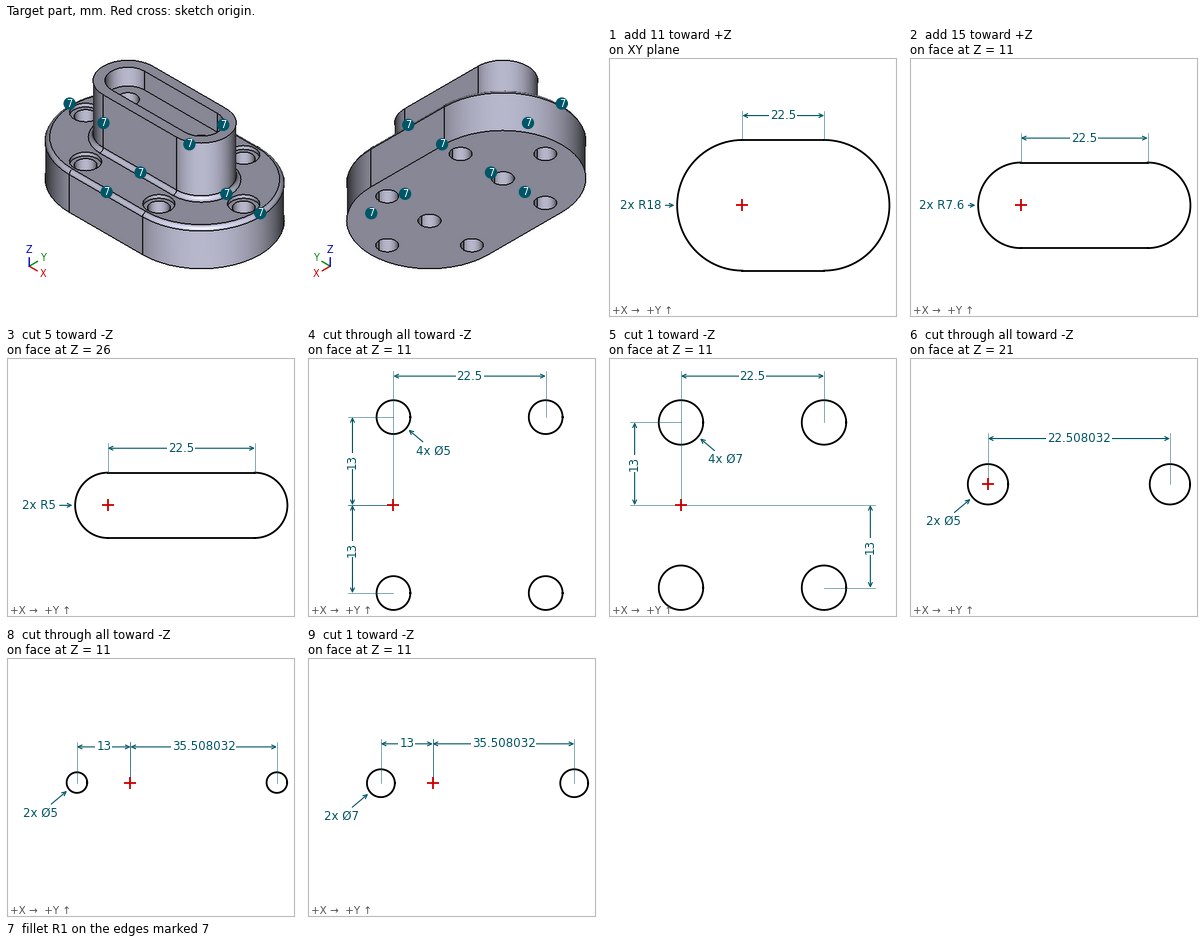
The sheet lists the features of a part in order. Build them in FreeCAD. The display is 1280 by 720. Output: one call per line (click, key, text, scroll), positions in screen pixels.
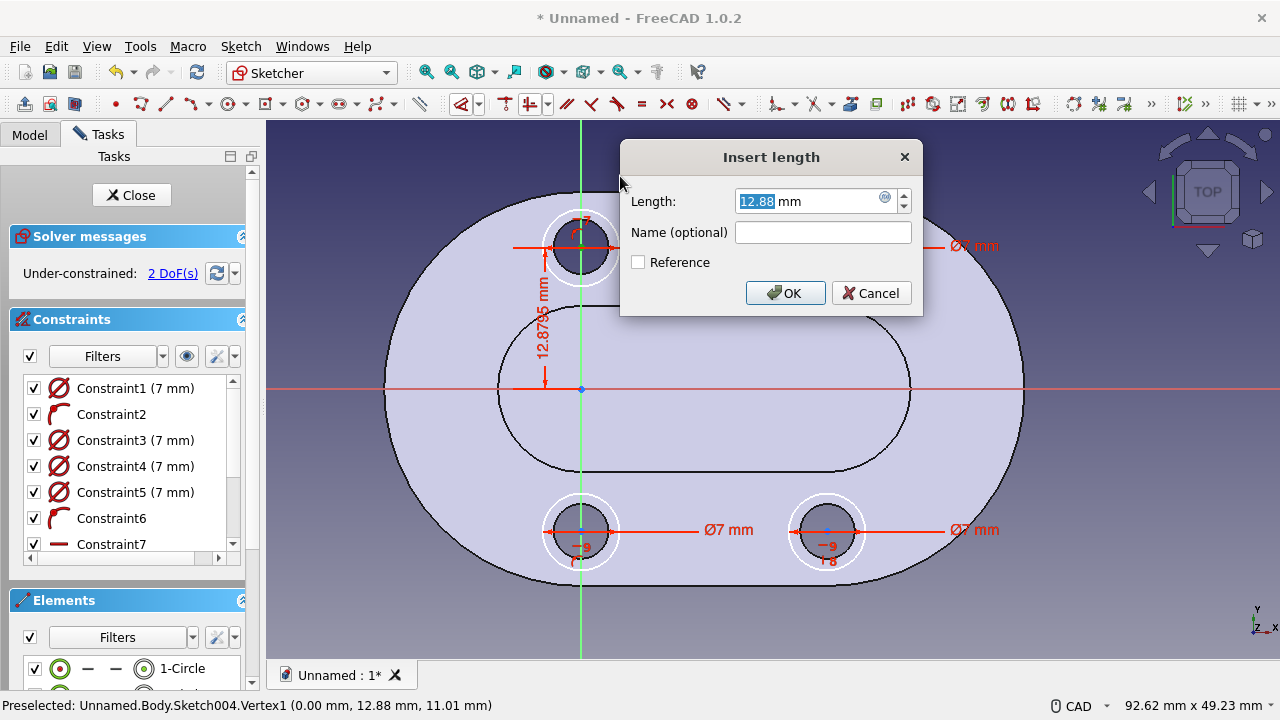
text(13)
key(Return)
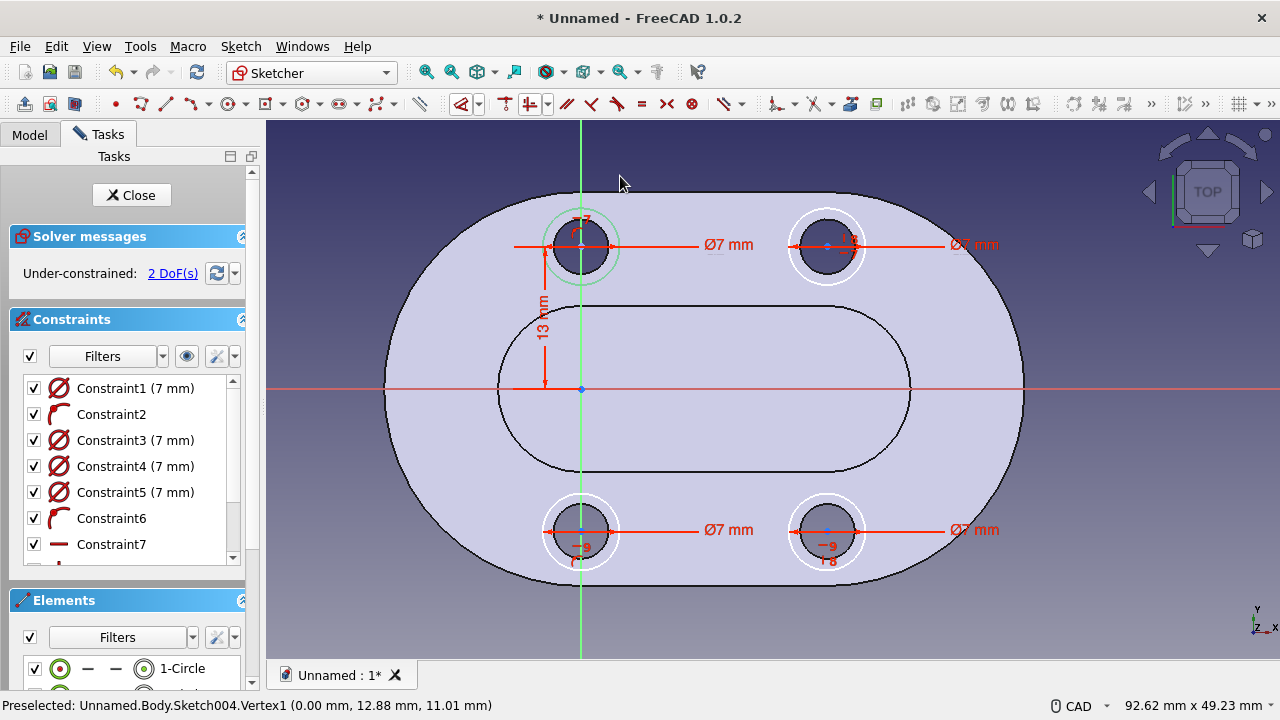
click(827, 532)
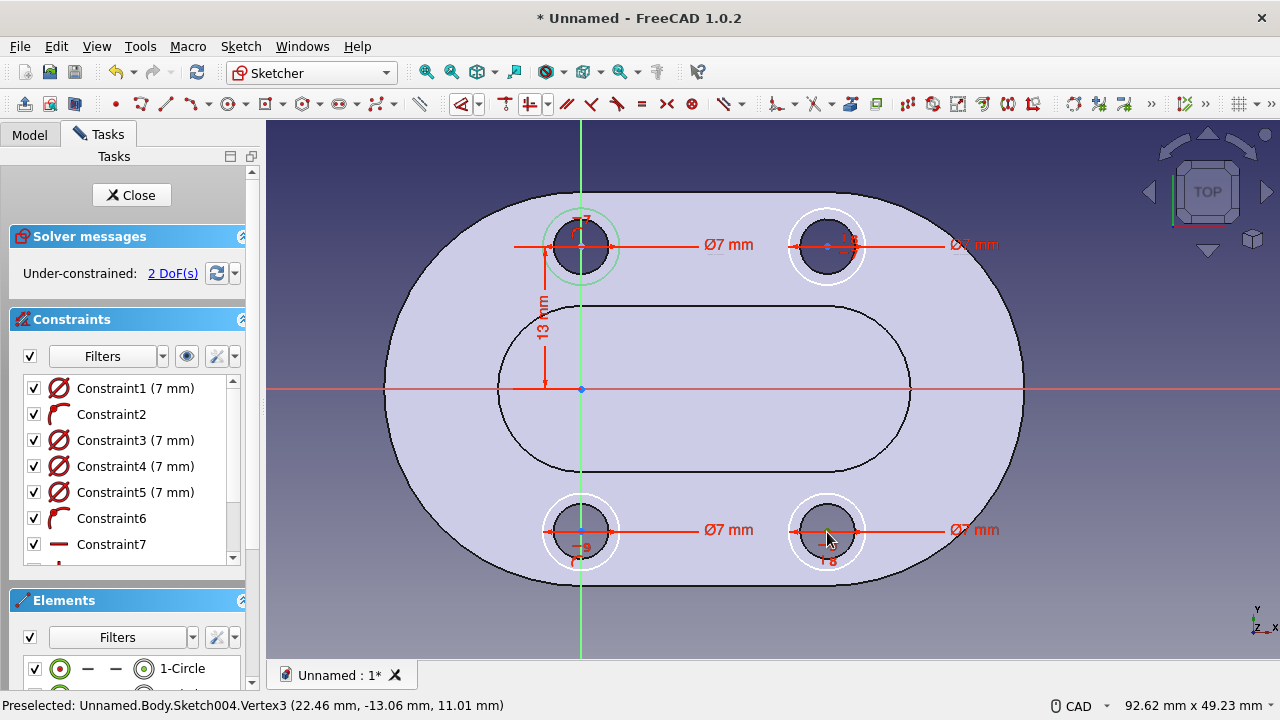
key(i)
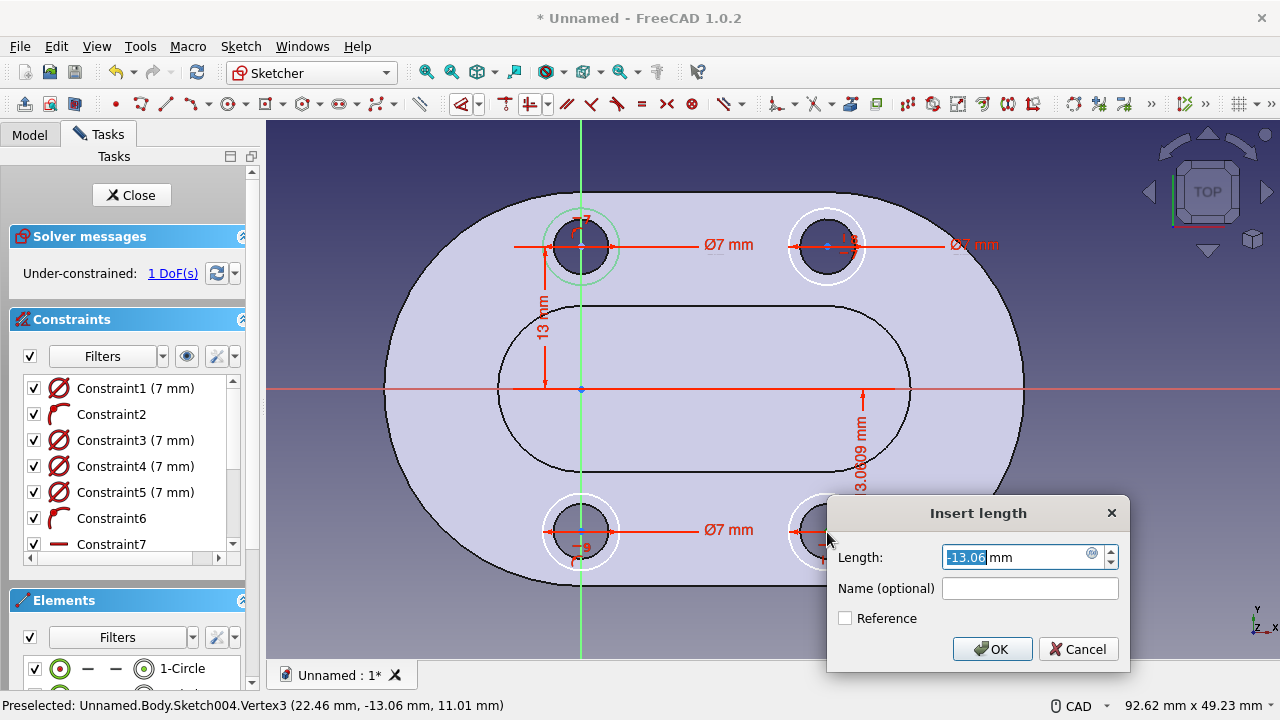
text(-13)
key(Return)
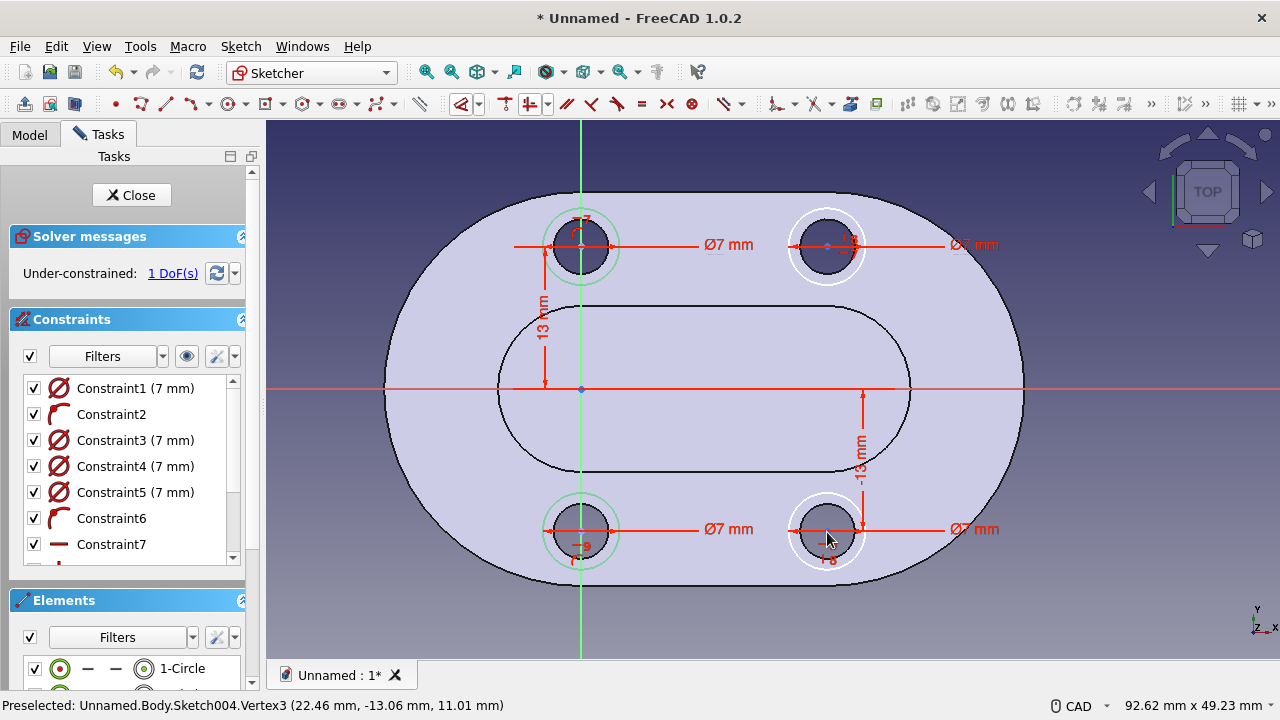
click(827, 247)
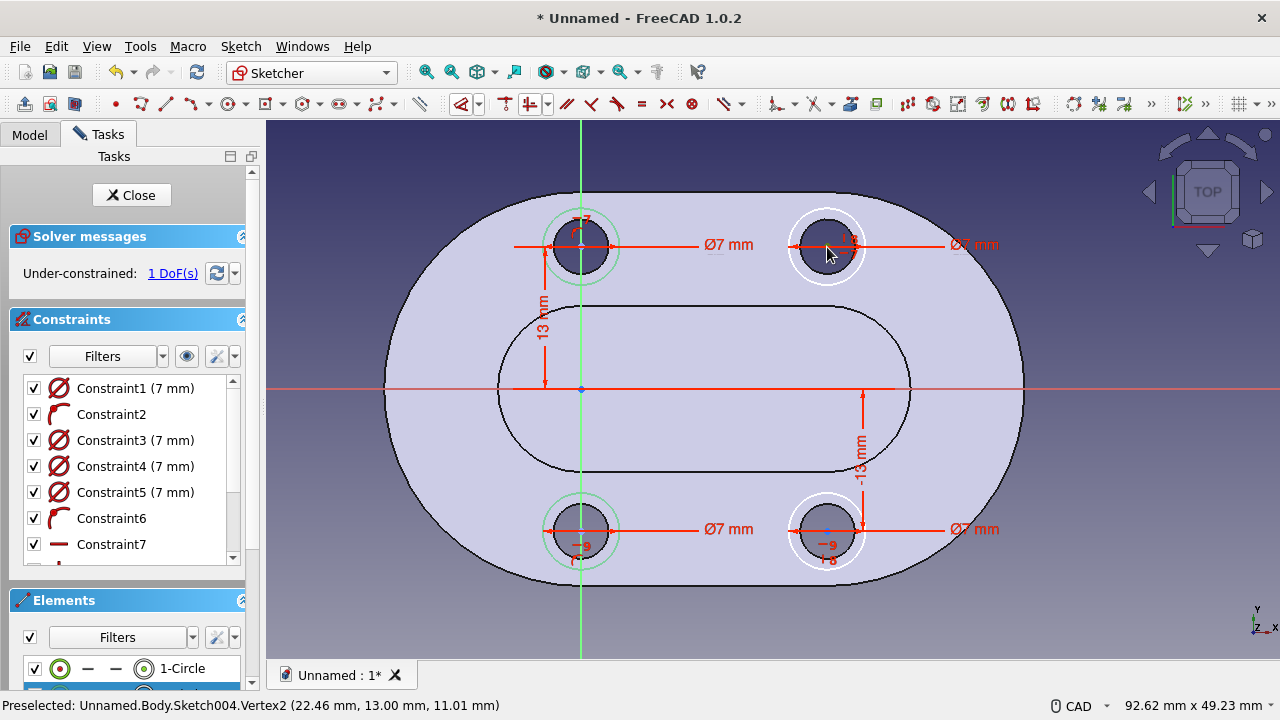
key(l)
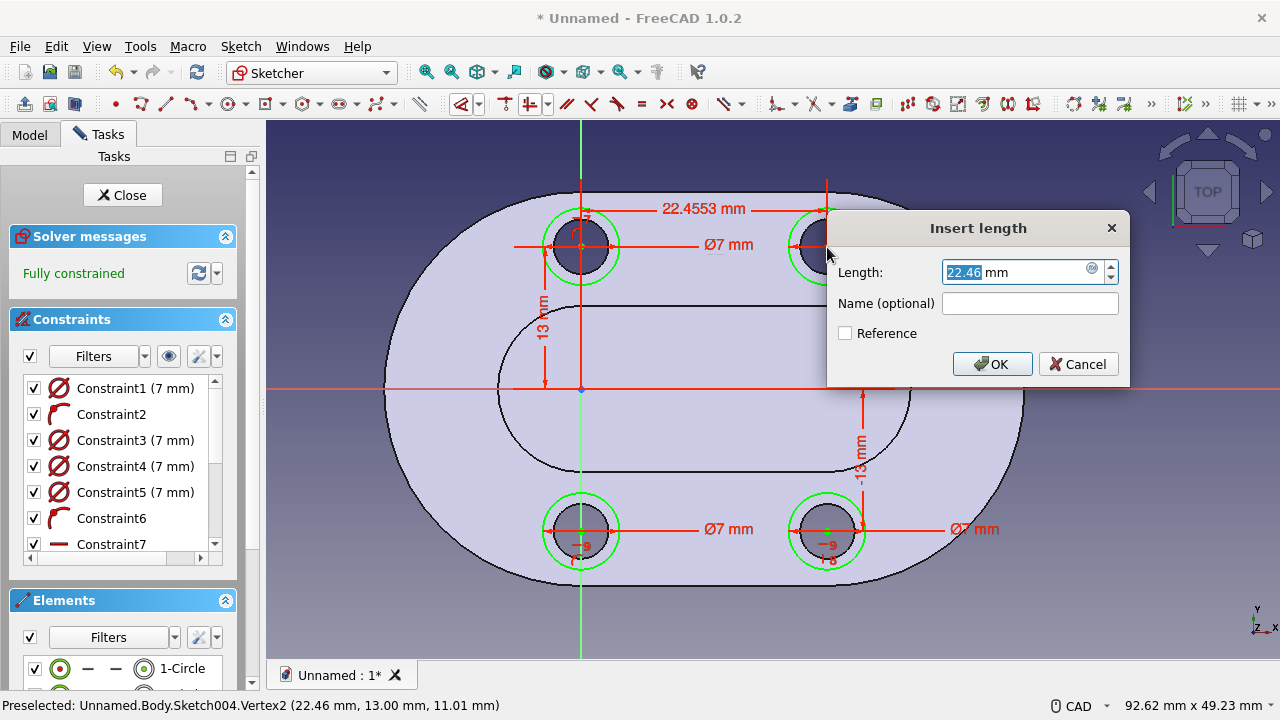
text(22.5)
key(Return)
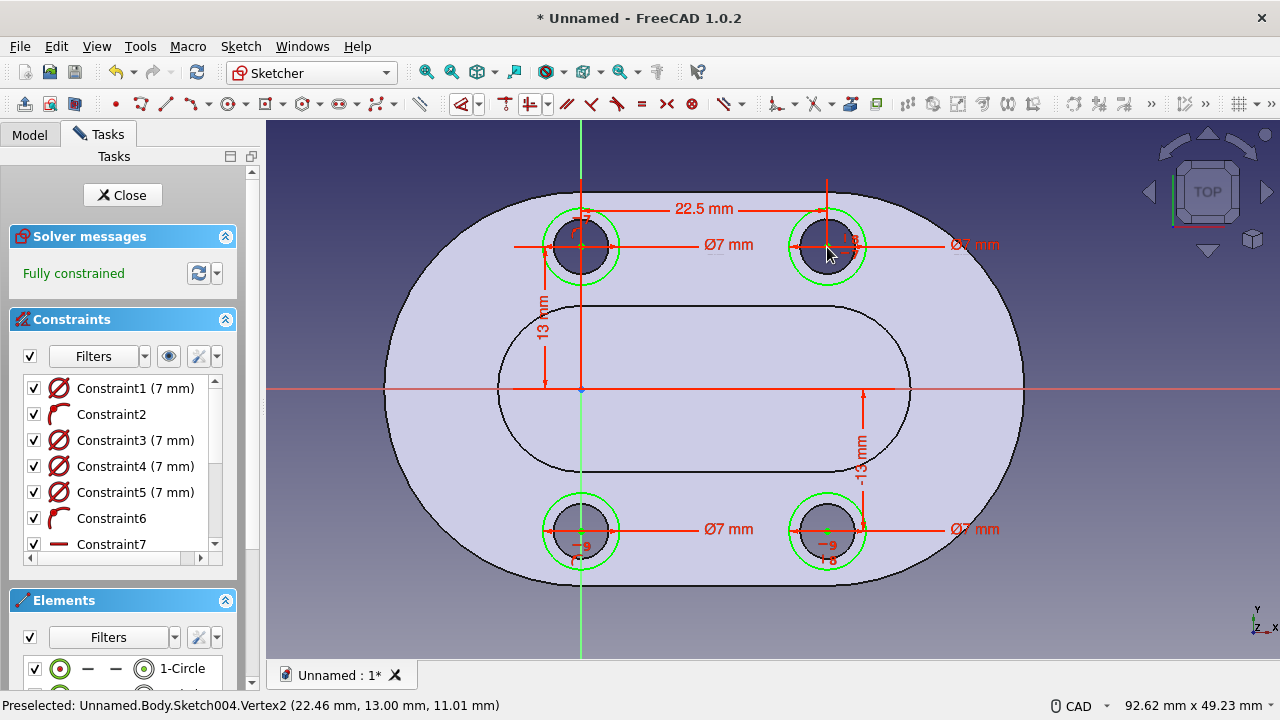
click(123, 195)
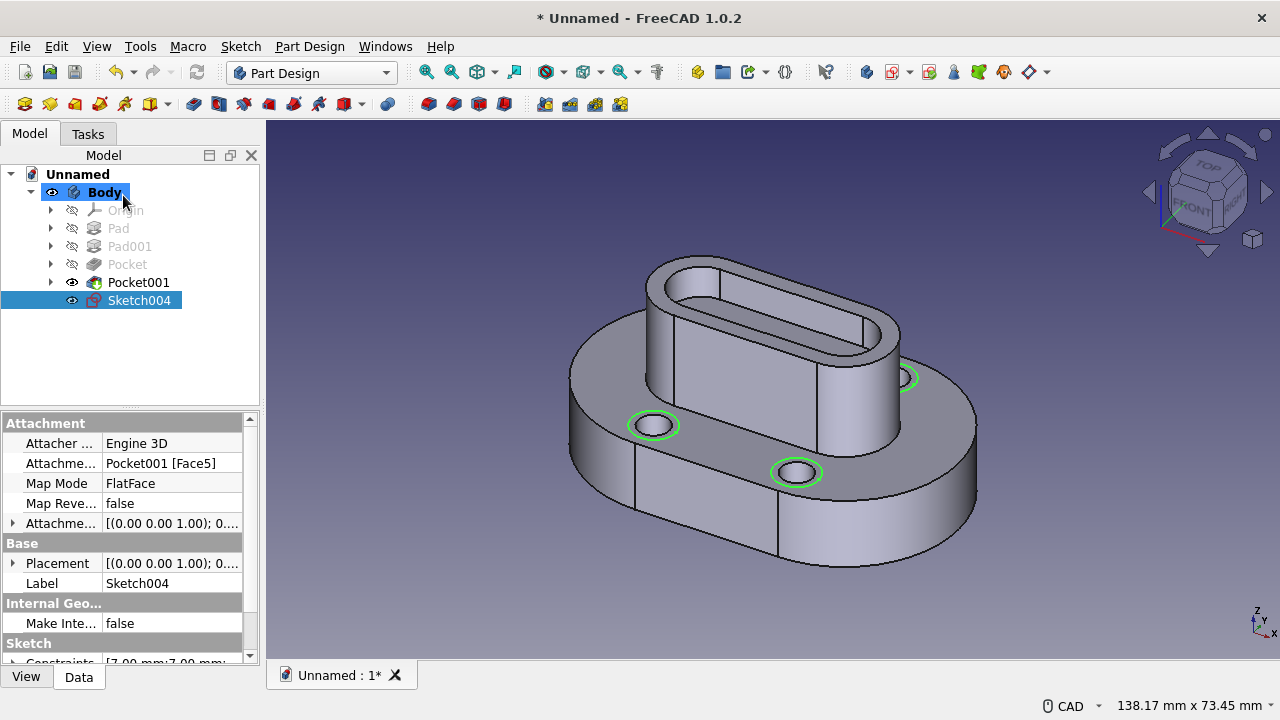
click(194, 104)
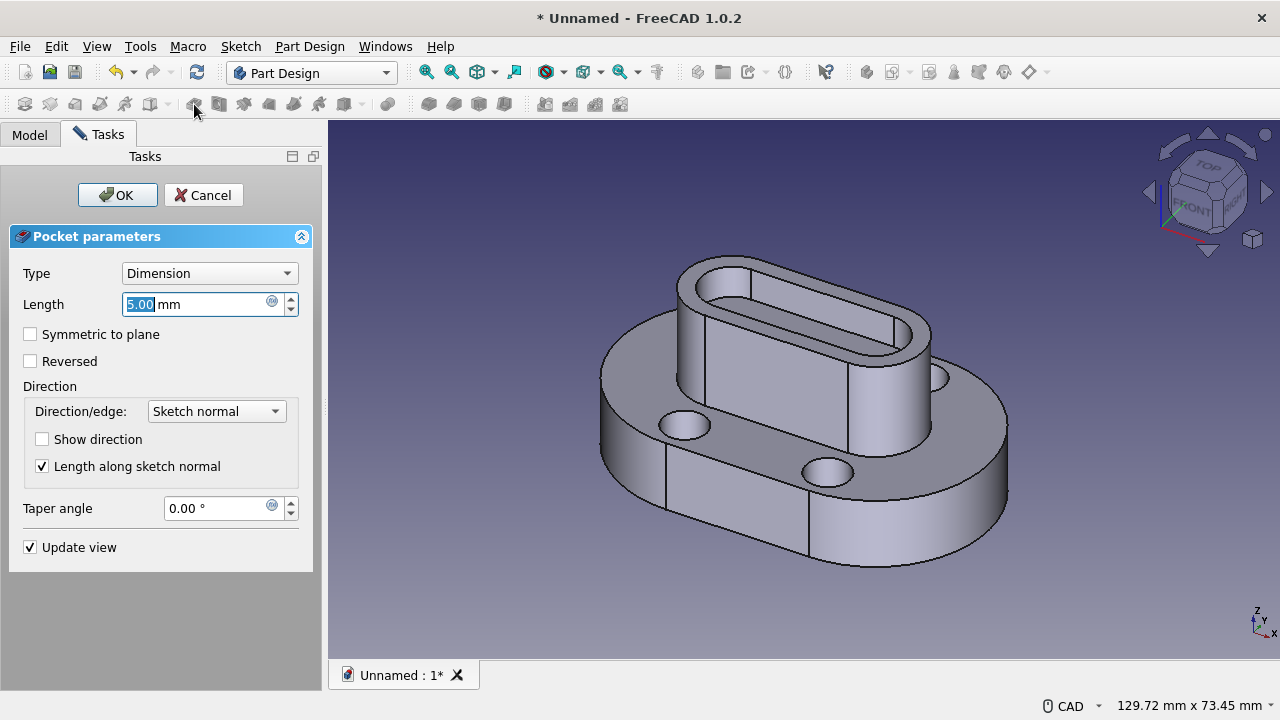
text(1)
key(Tab)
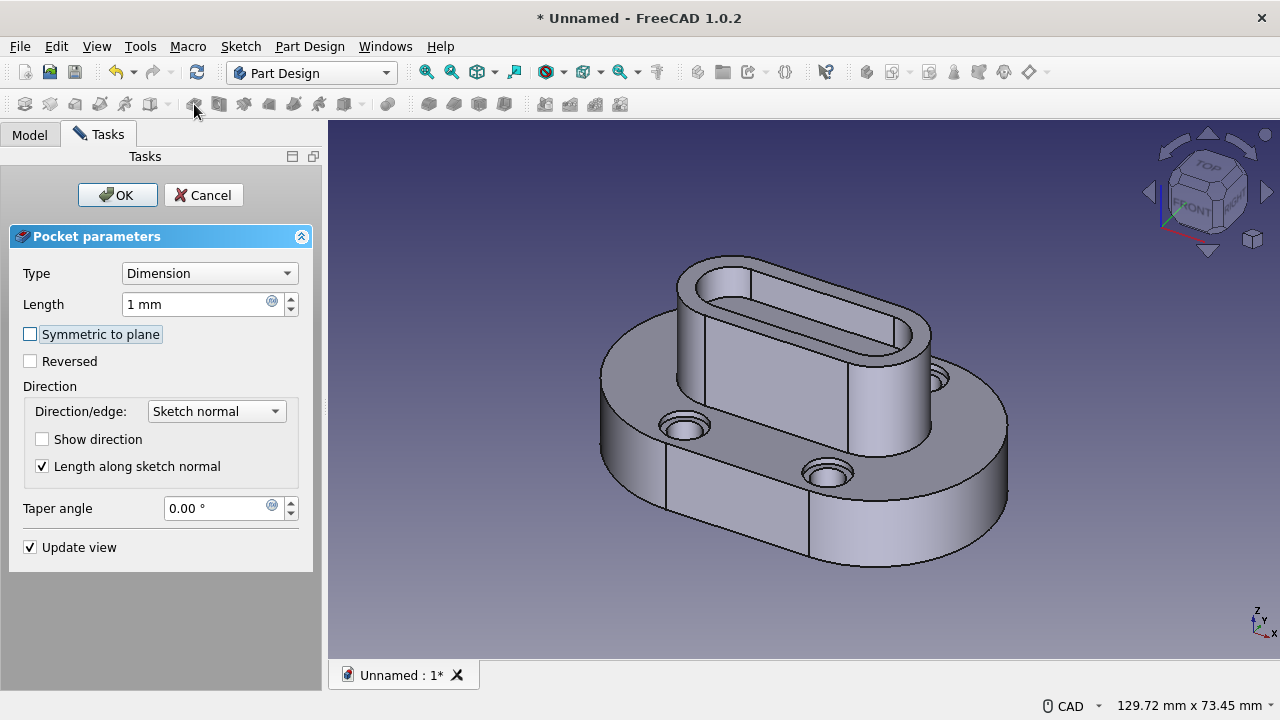
click(118, 195)